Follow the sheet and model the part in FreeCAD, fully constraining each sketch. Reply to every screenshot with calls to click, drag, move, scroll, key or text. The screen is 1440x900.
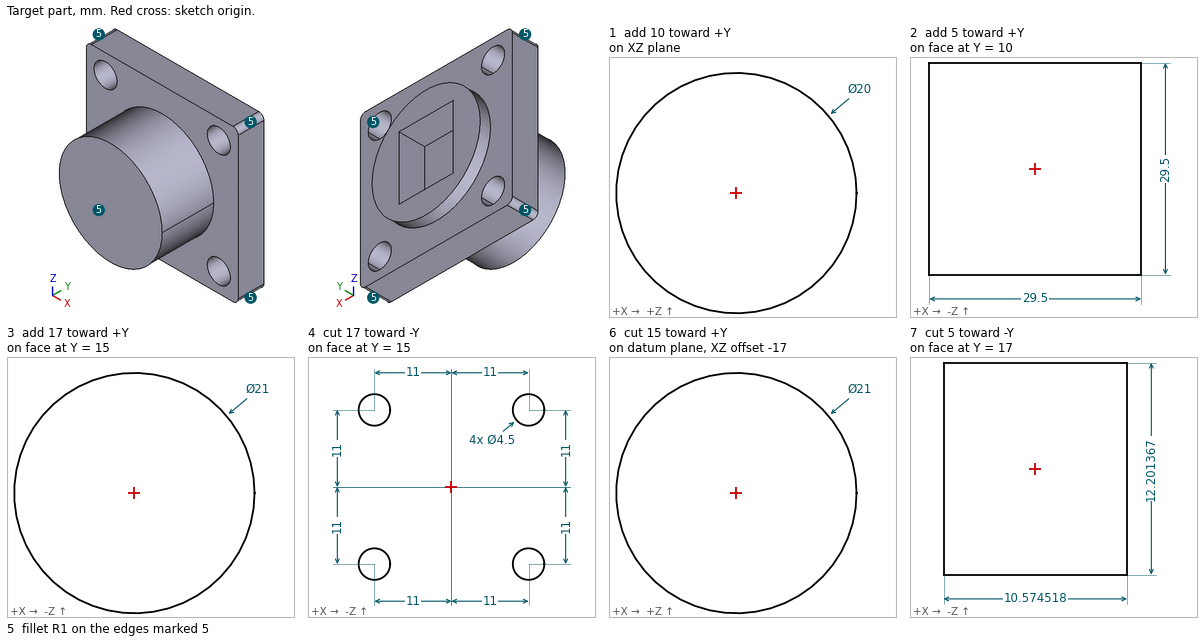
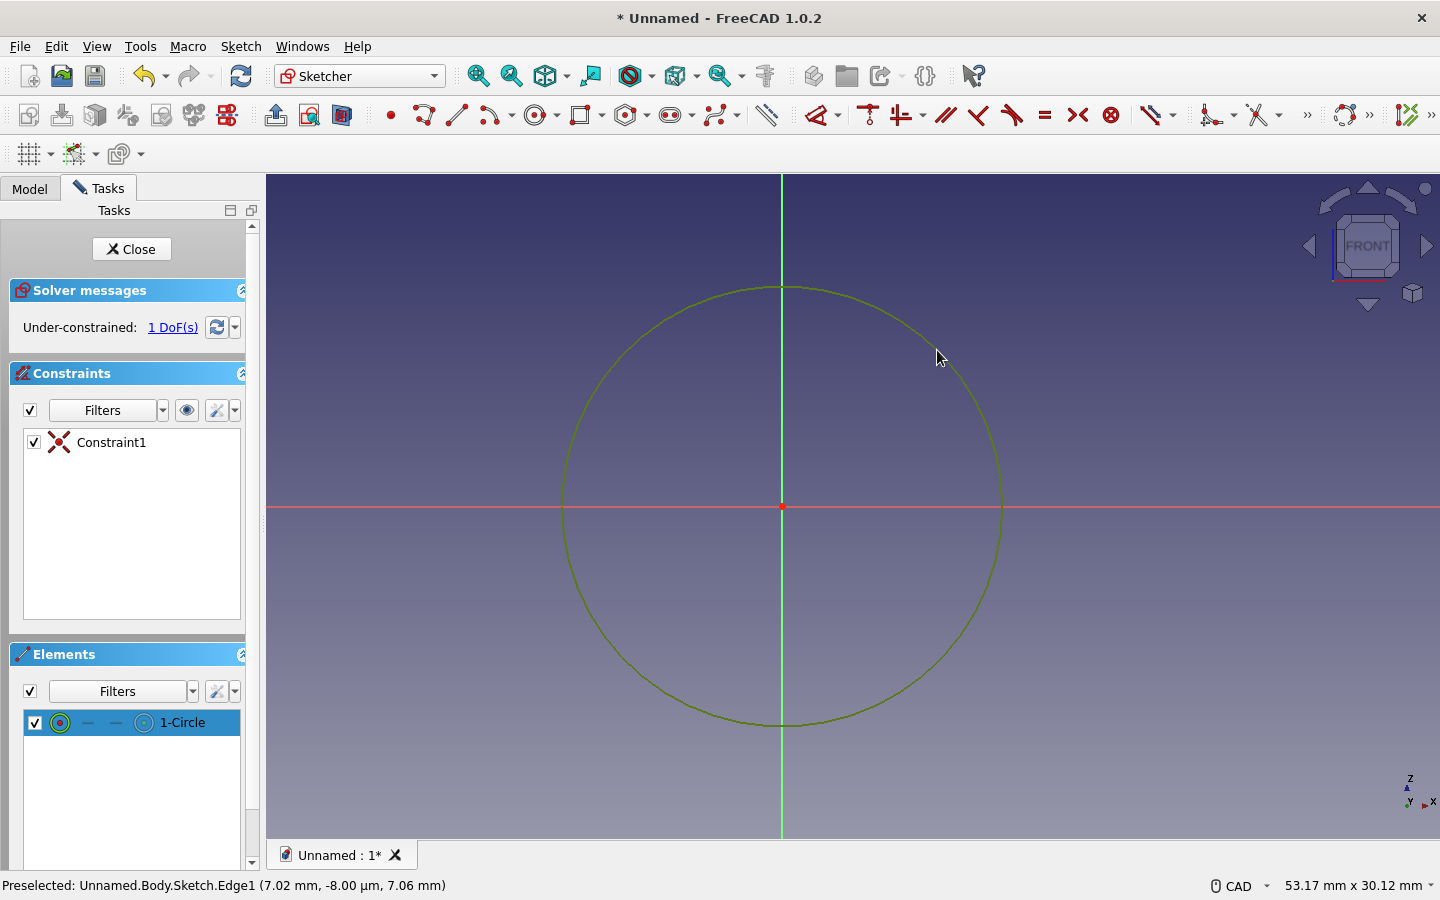
click(838, 116)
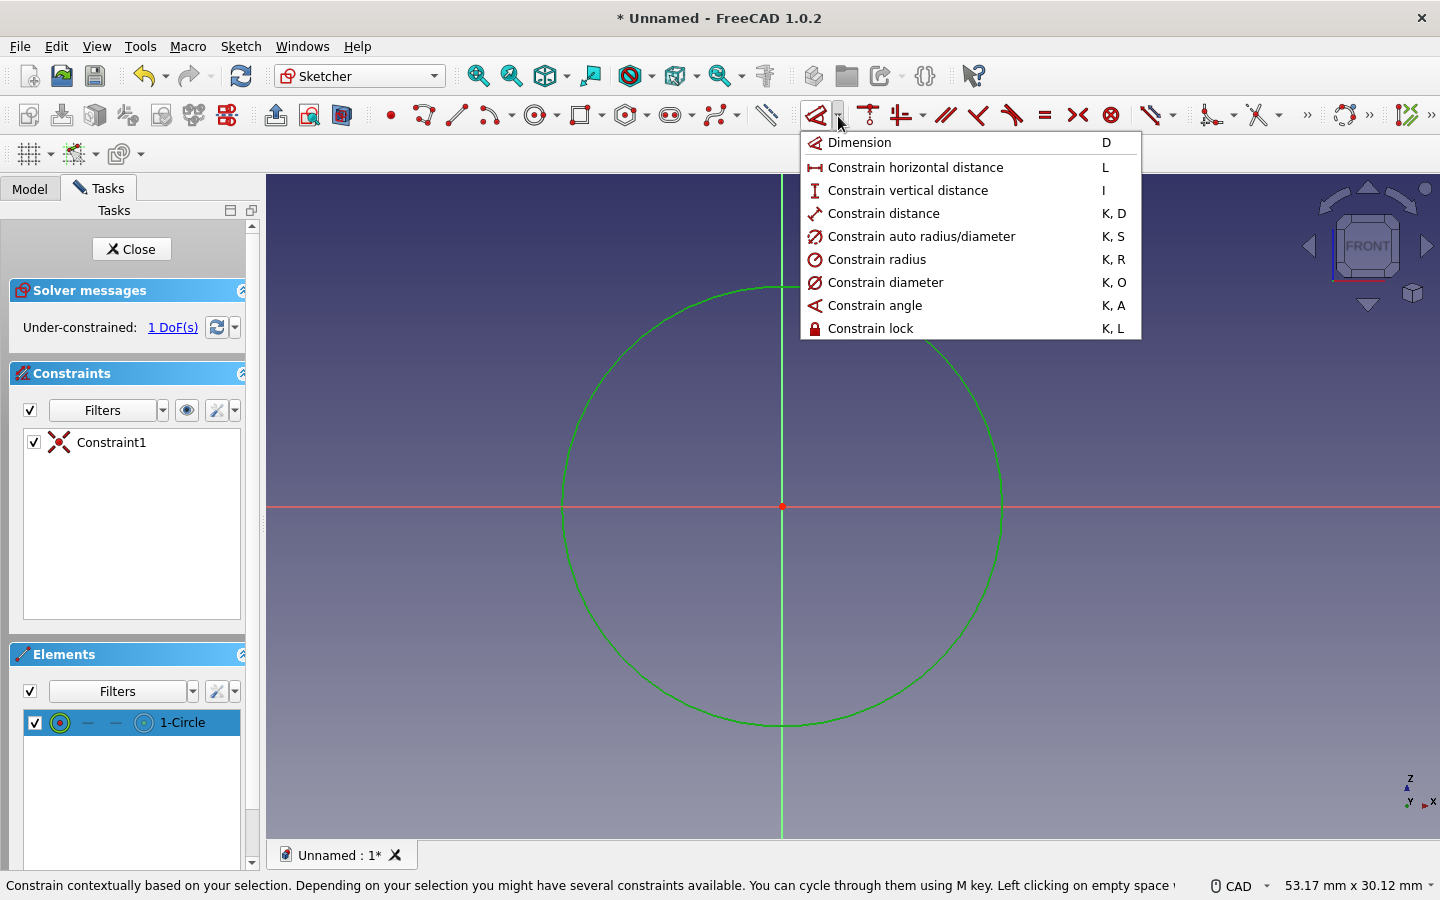
click(971, 282)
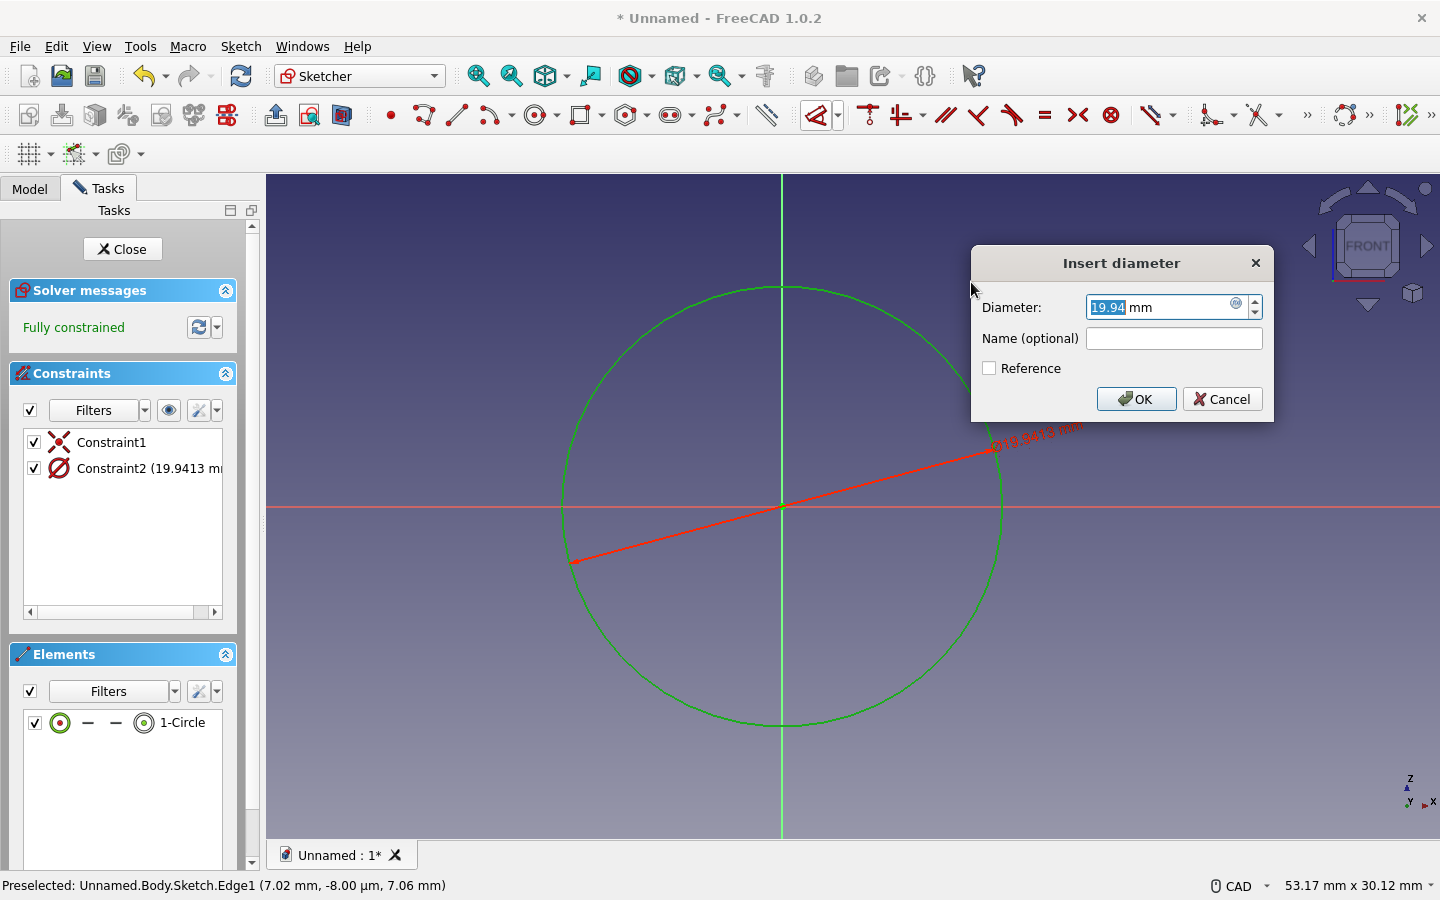
text(20)
key(Return)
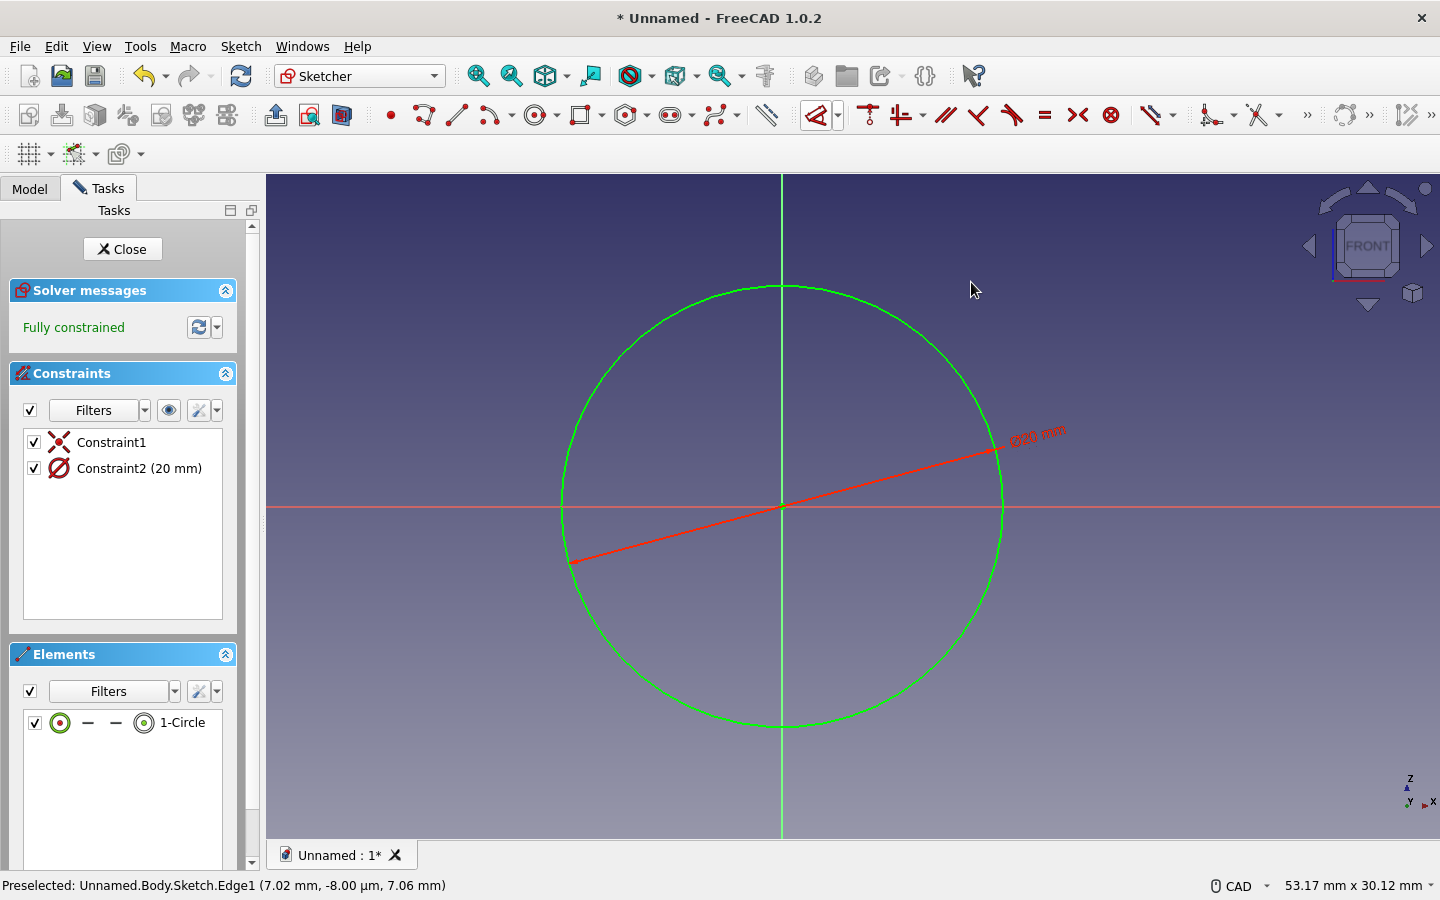
click(123, 249)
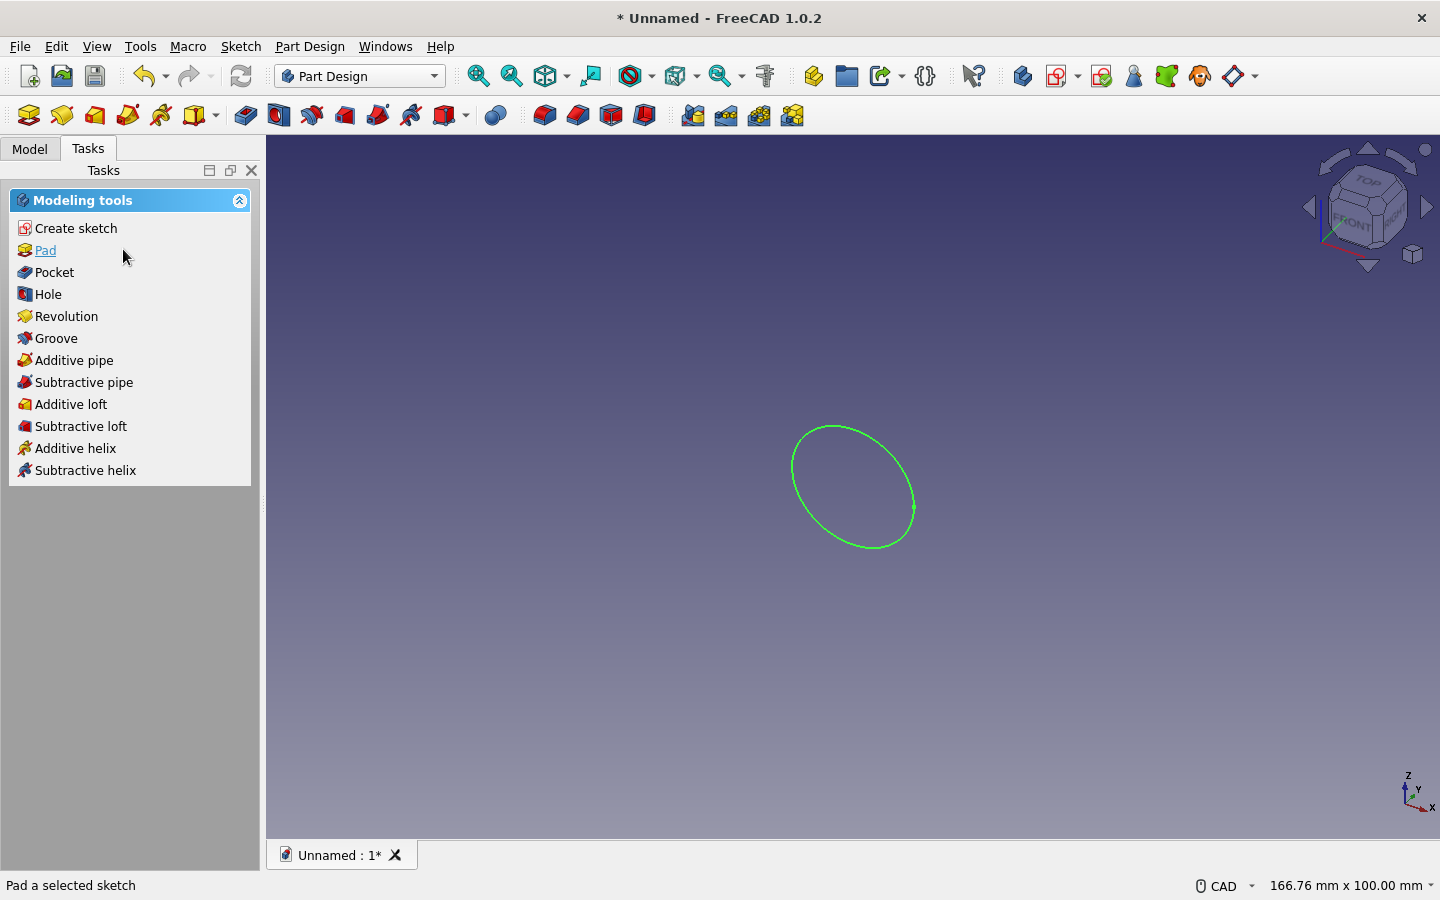
click(29, 116)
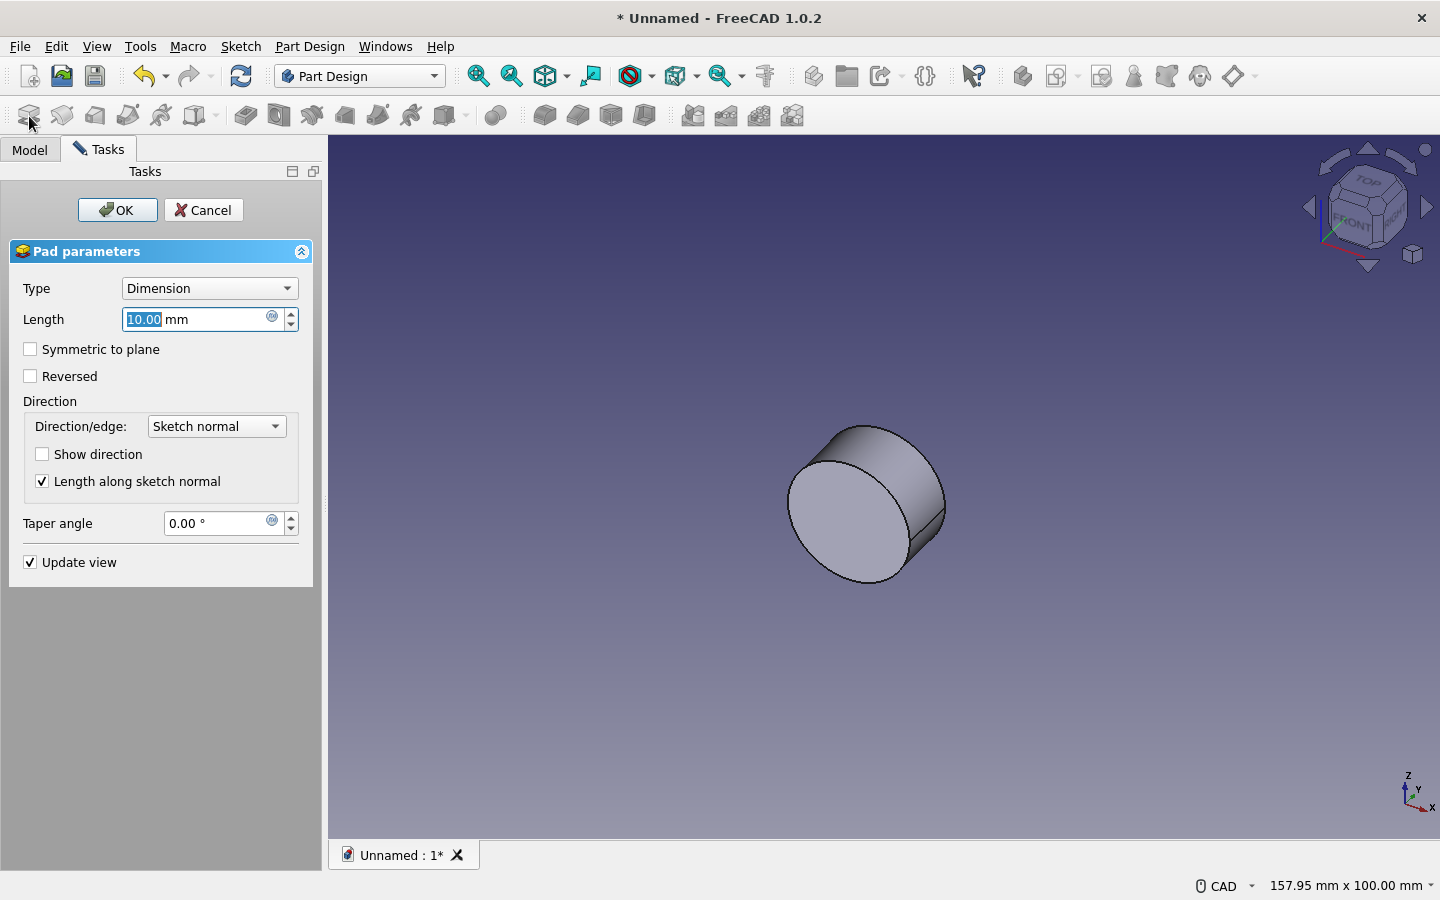
text(10)
key(Tab)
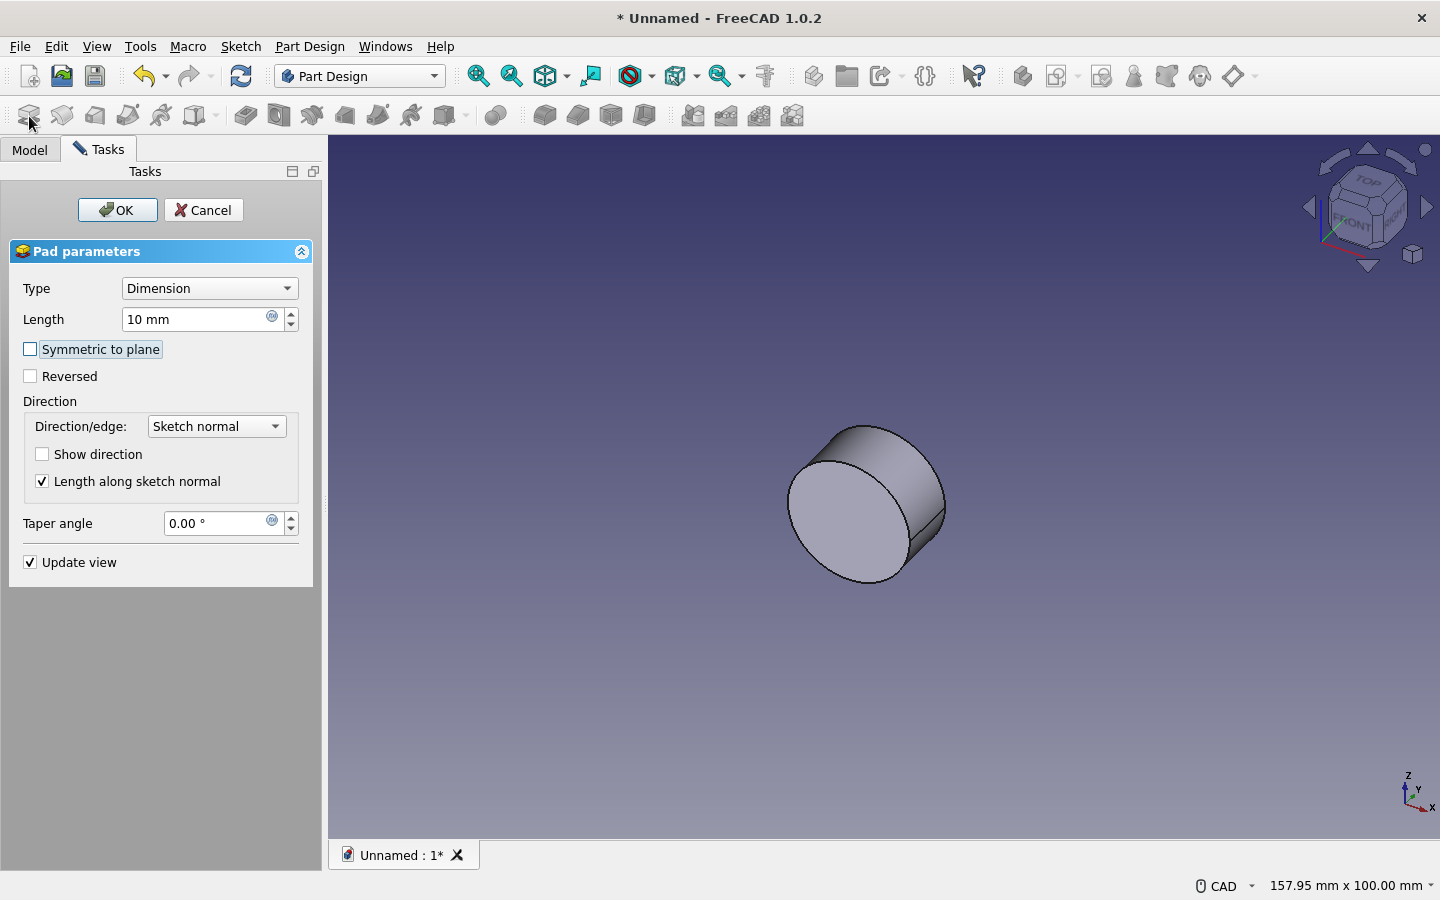
click(31, 376)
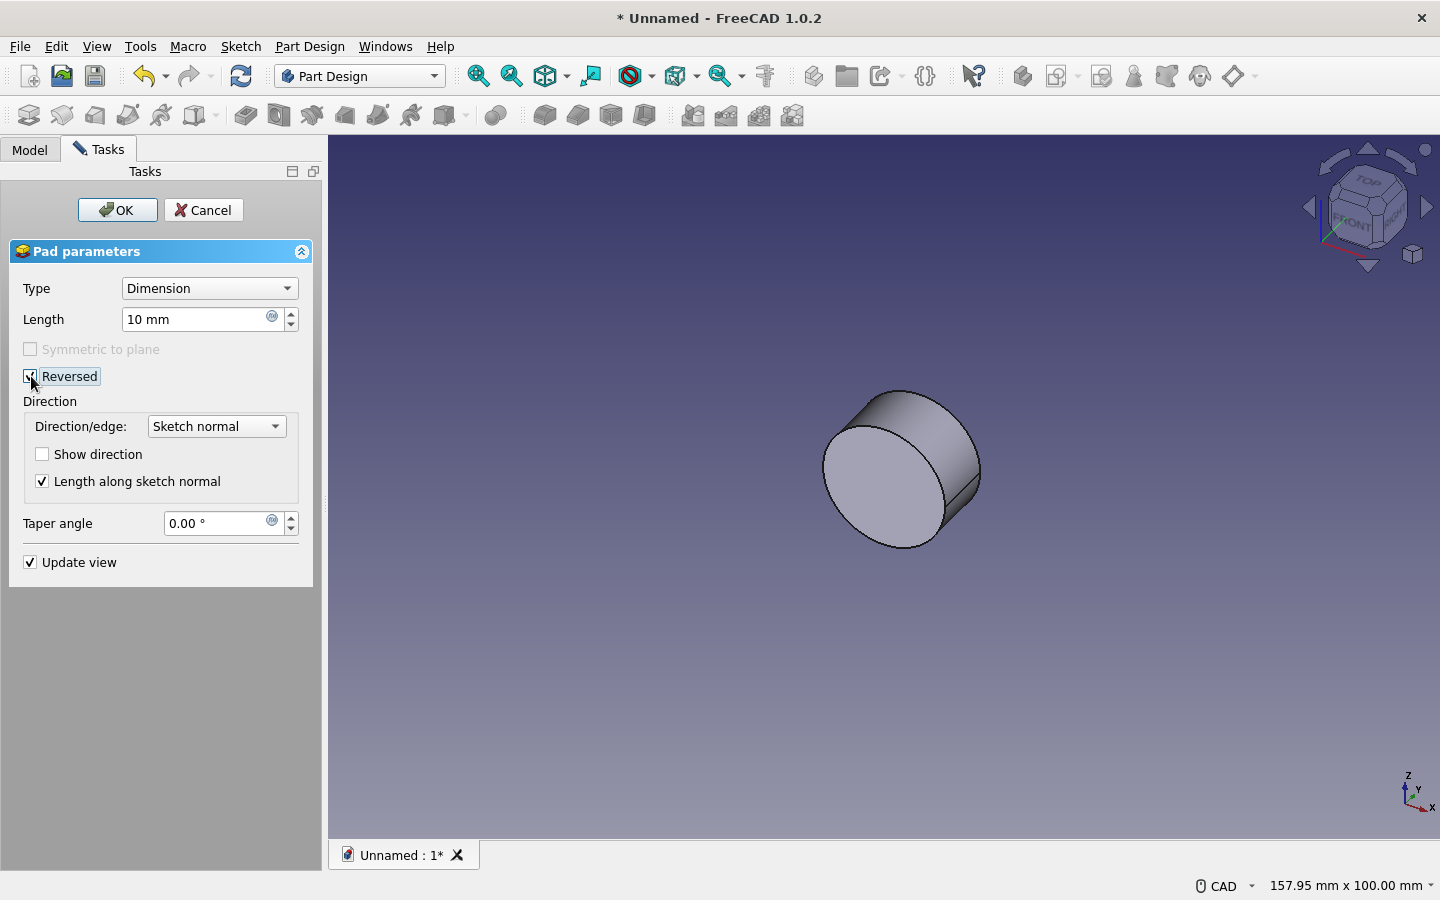
click(118, 210)